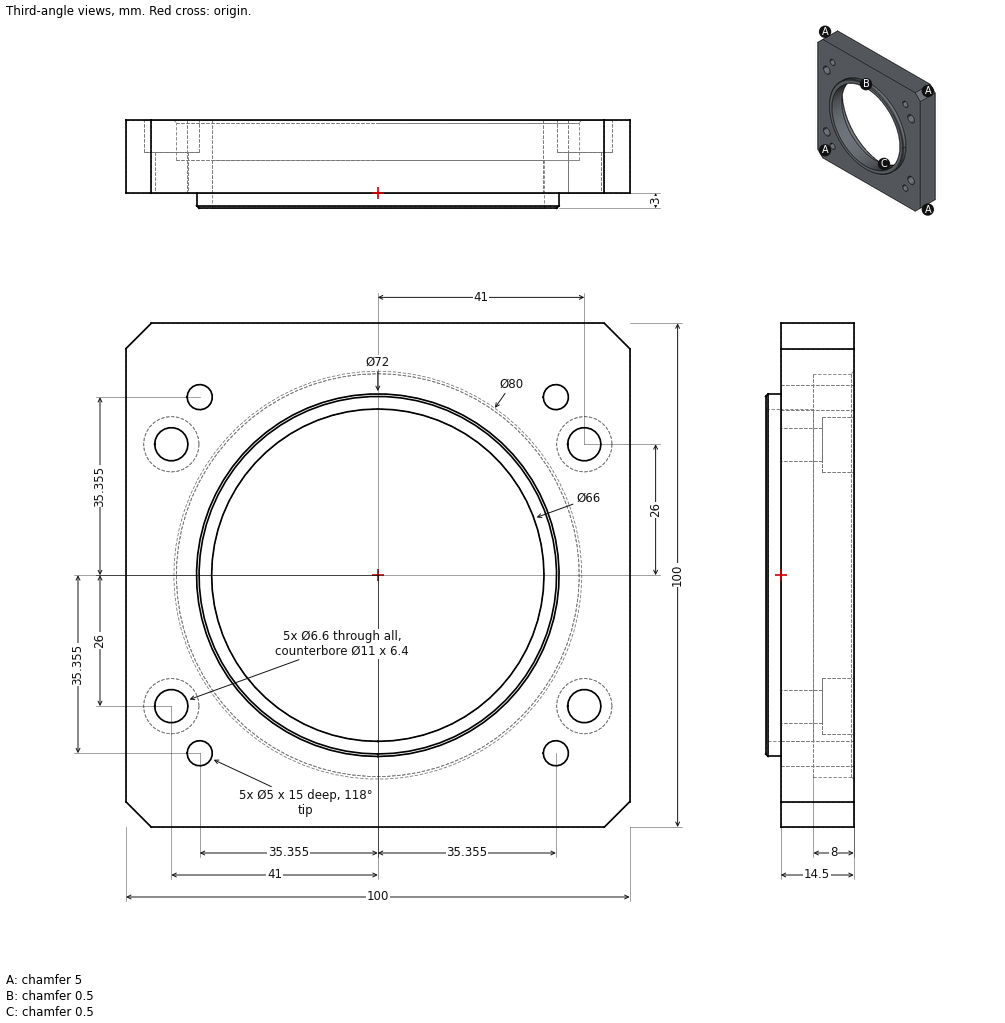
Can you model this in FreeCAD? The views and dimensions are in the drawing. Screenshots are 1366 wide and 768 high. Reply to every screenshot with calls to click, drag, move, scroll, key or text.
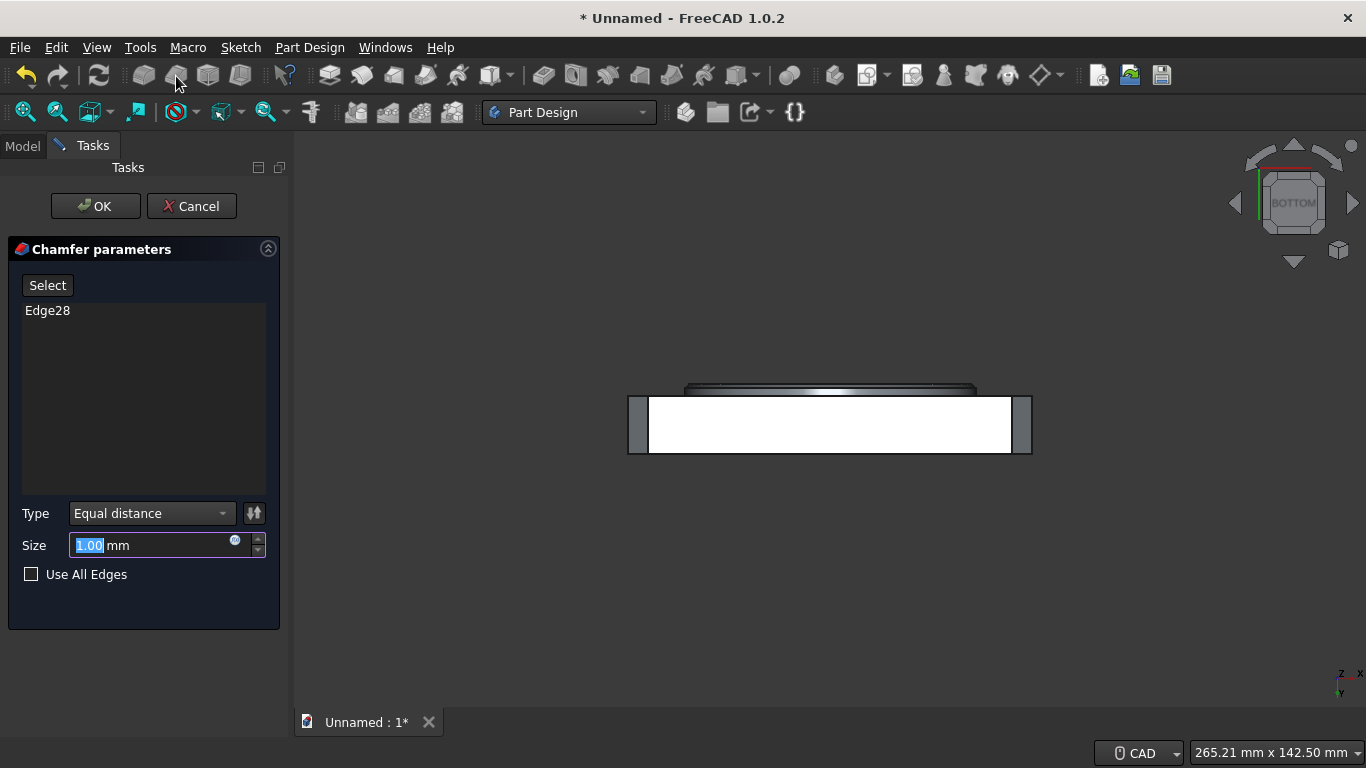
text(0.5)
key(Tab)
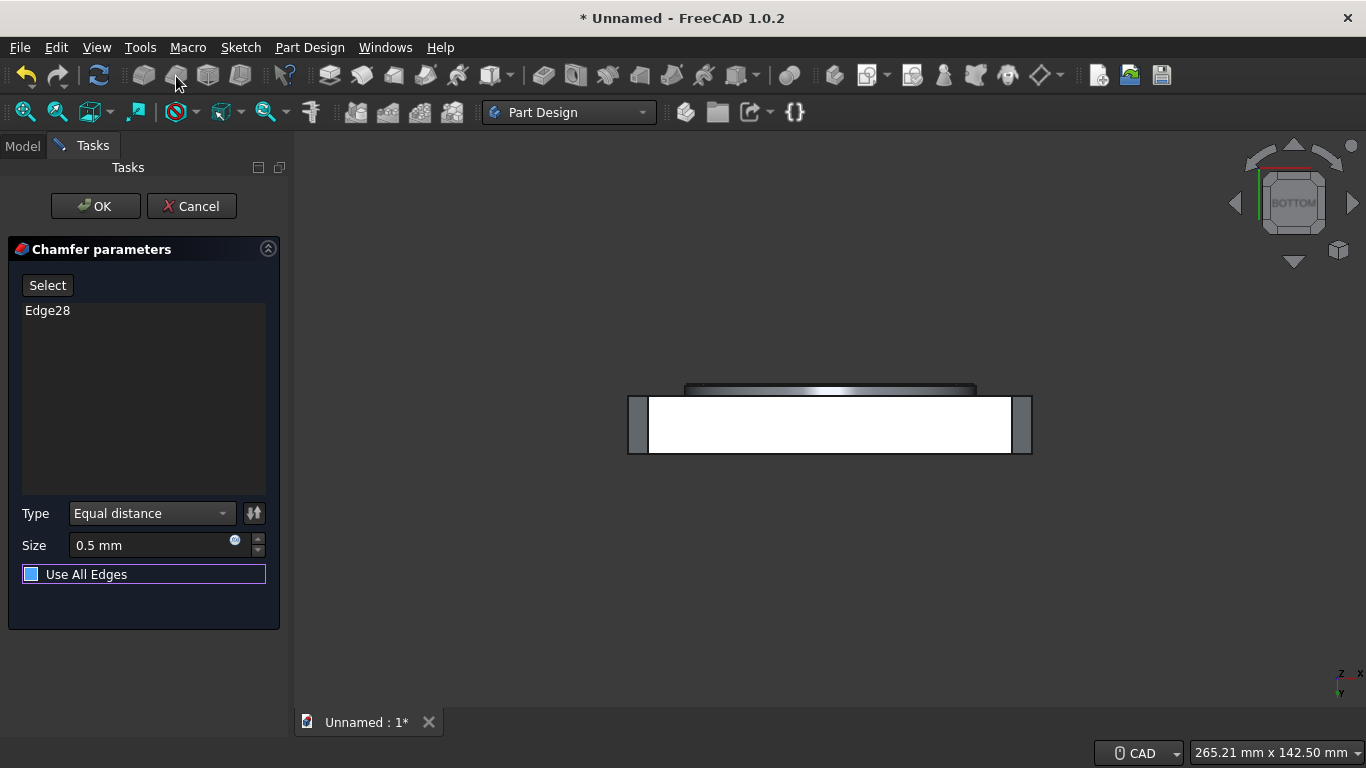
click(96, 206)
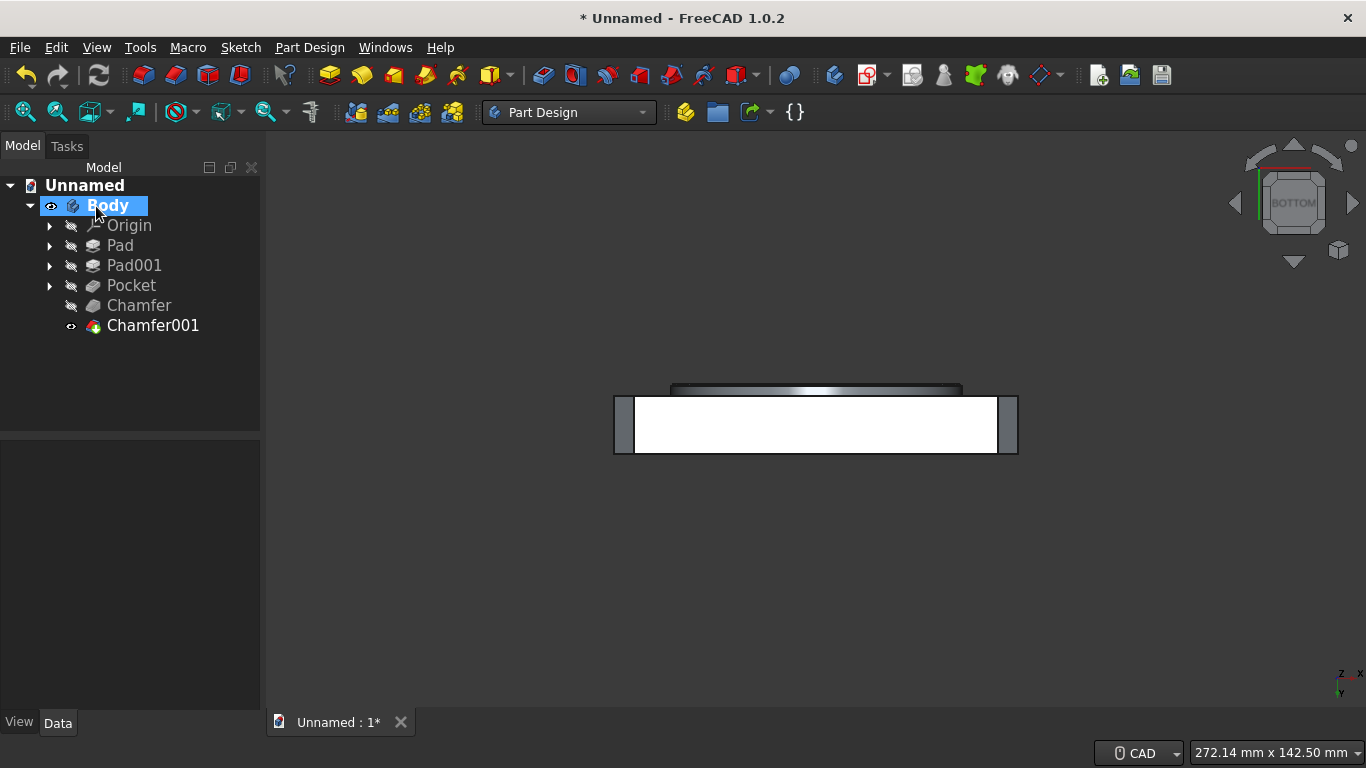
key(v)
key(f)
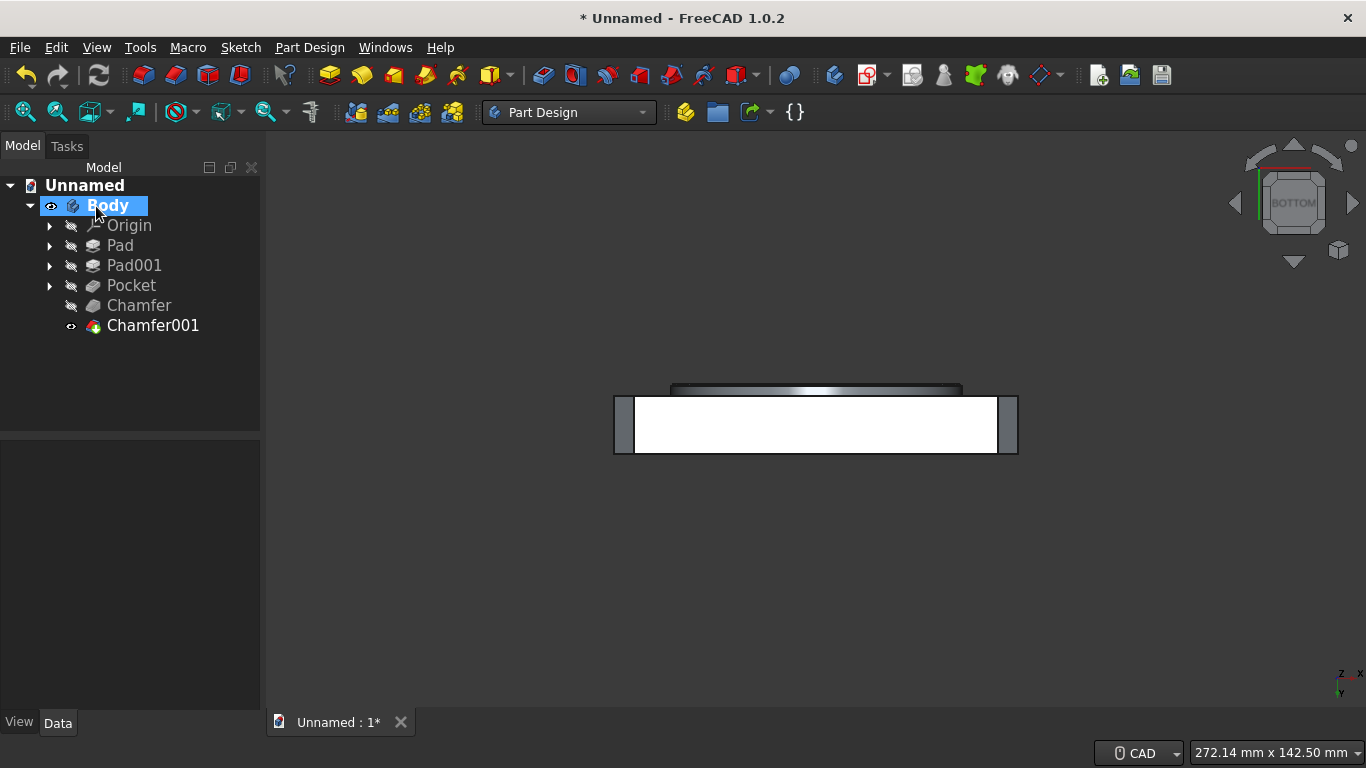
key(4)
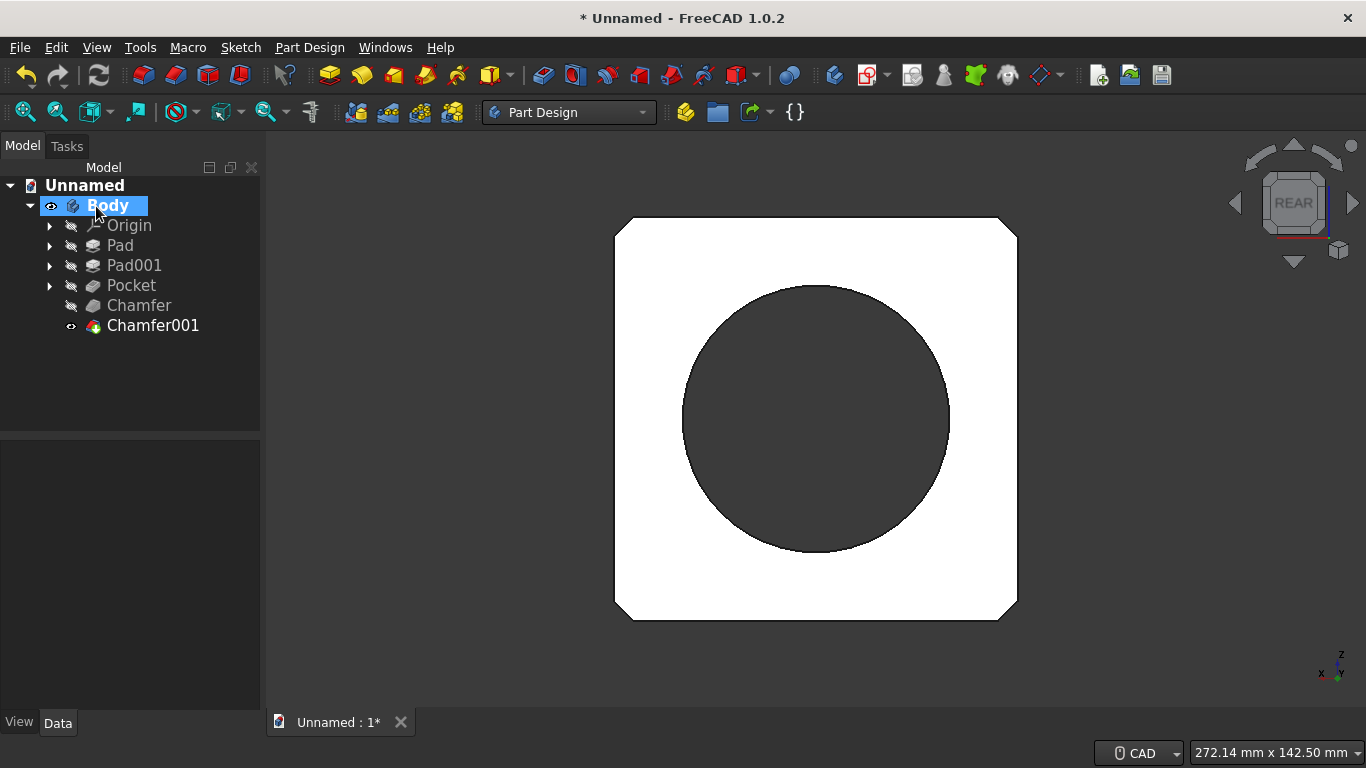
click(701, 533)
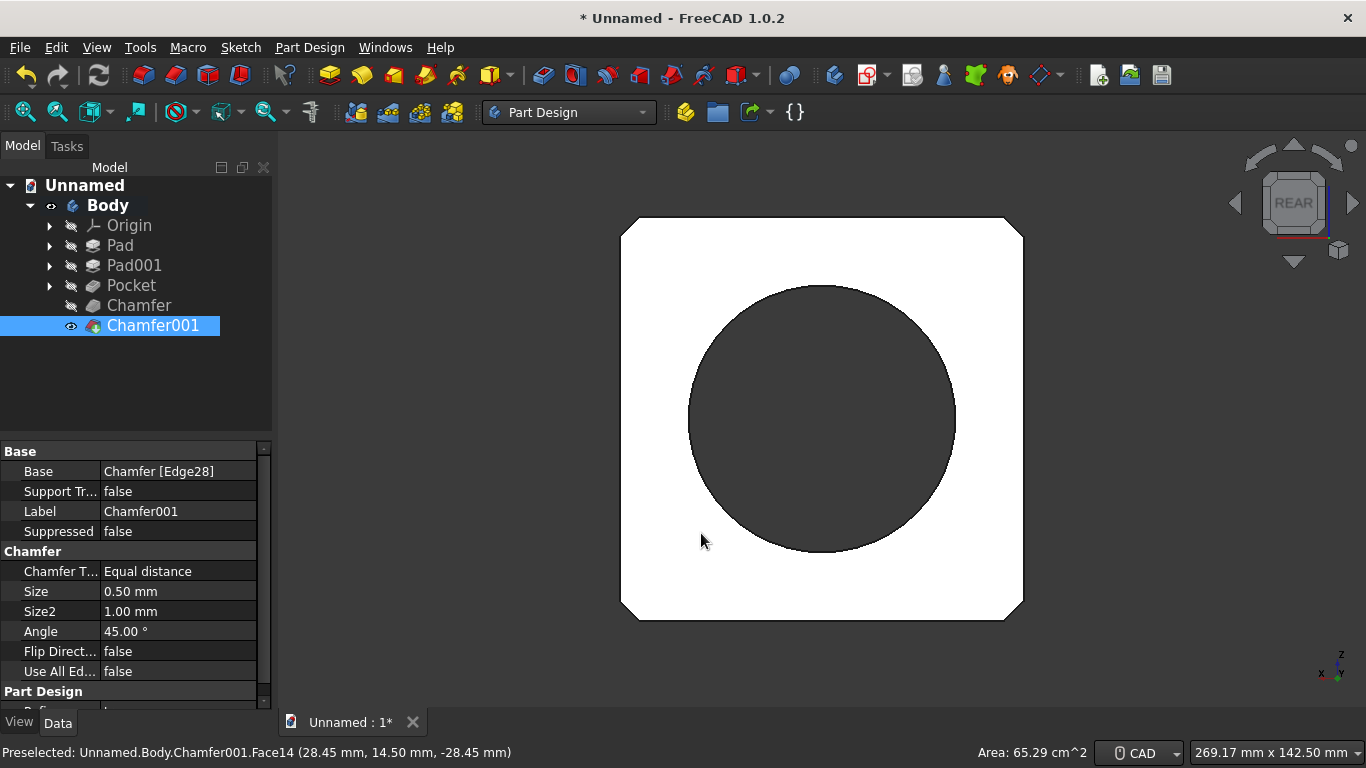
click(868, 76)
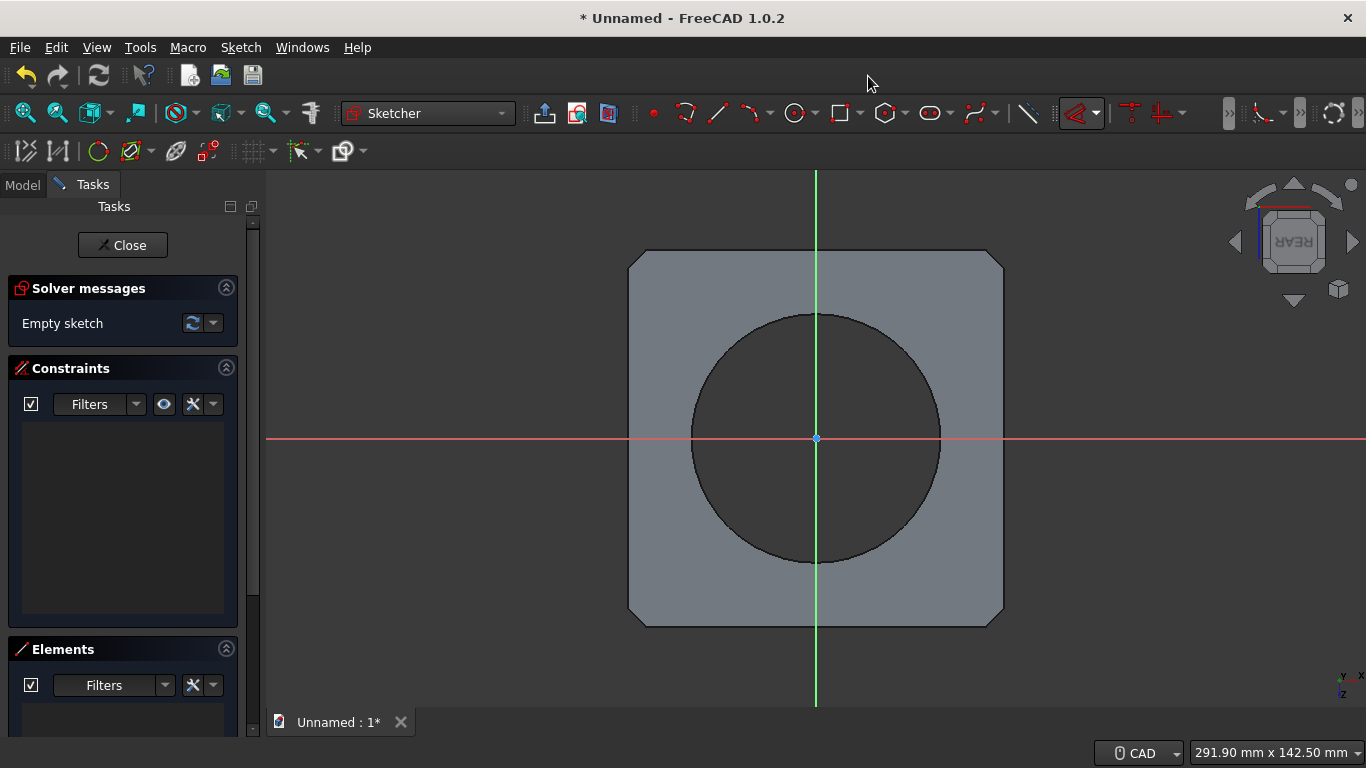
key(g)
key(c)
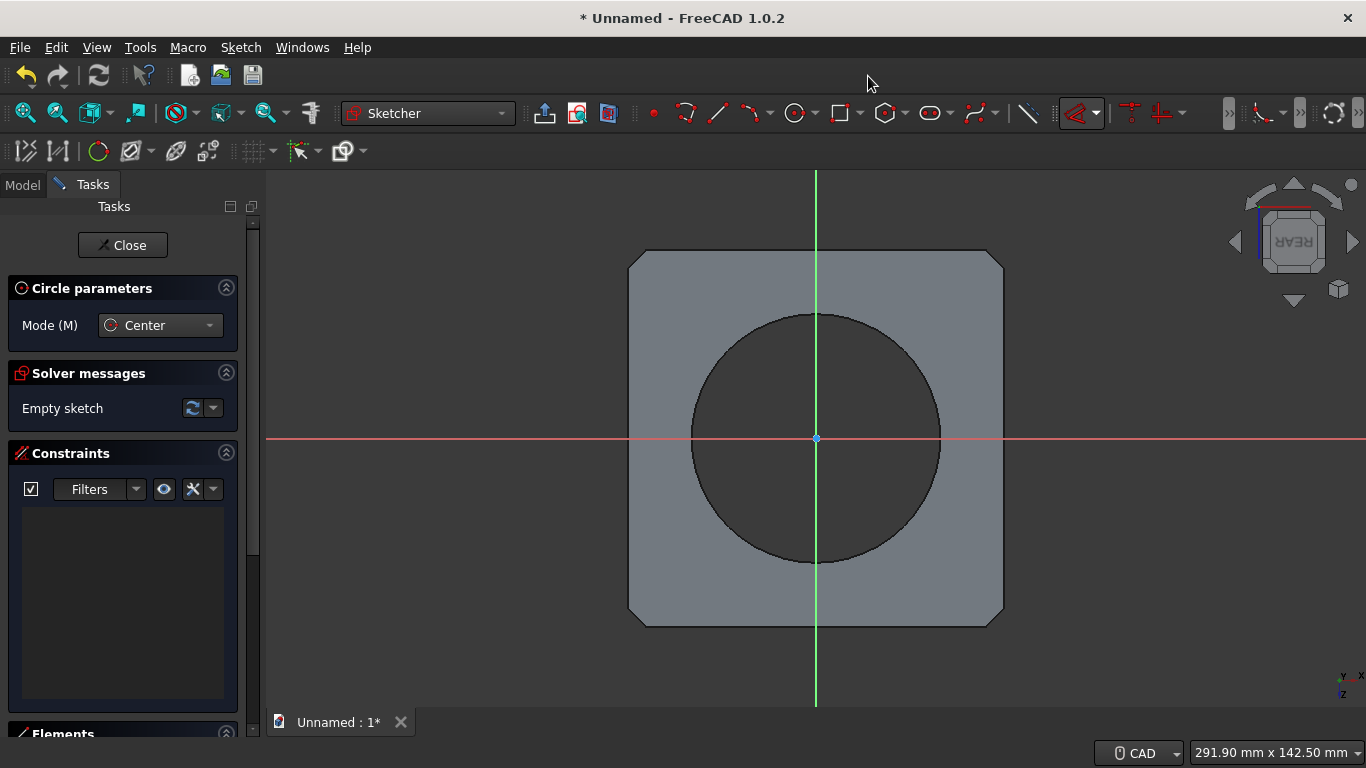
click(816, 439)
click(923, 332)
key(Escape)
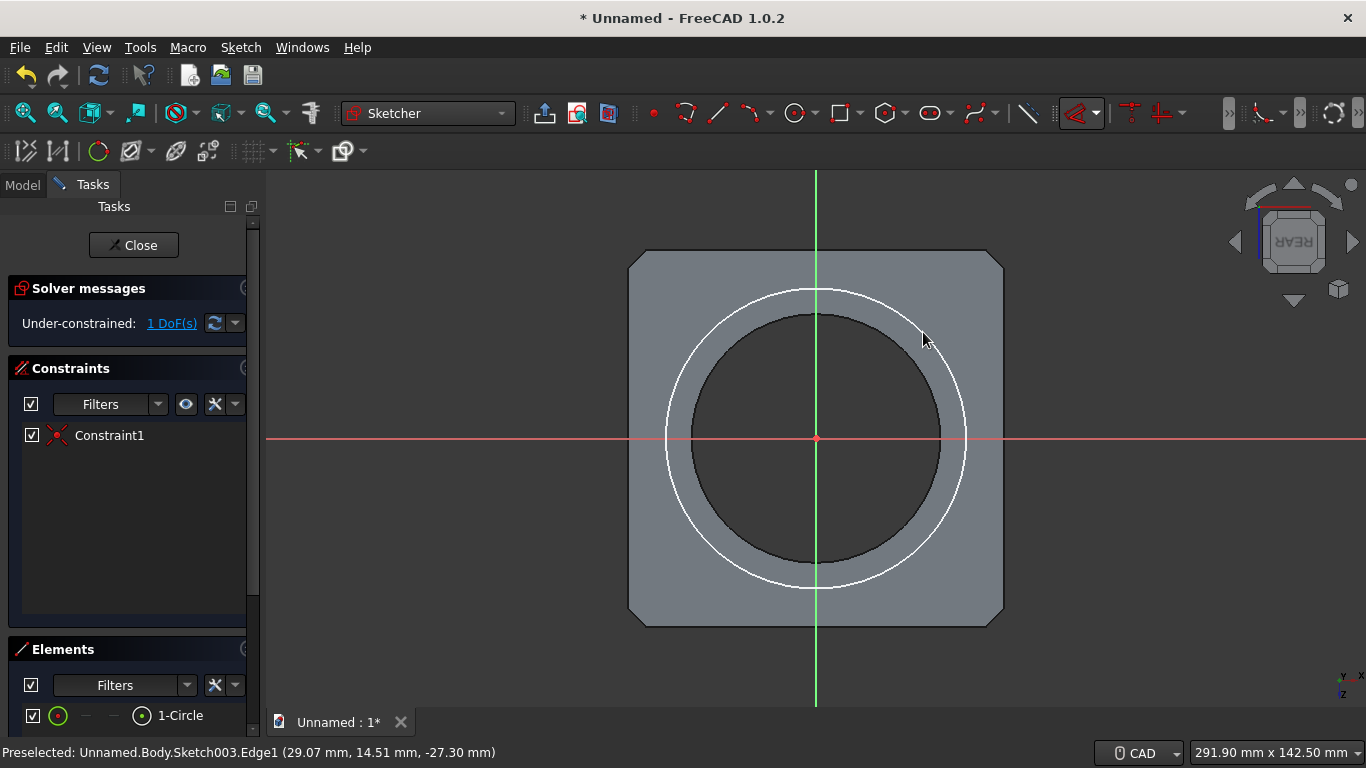
key(d)